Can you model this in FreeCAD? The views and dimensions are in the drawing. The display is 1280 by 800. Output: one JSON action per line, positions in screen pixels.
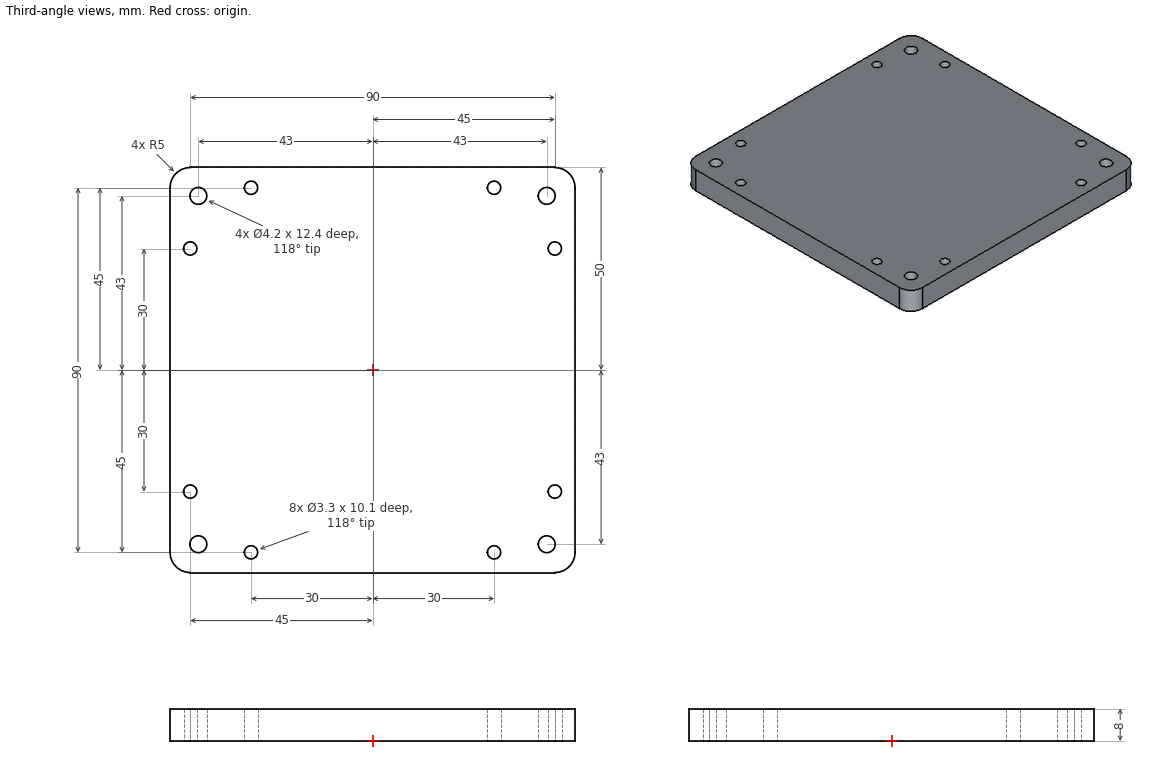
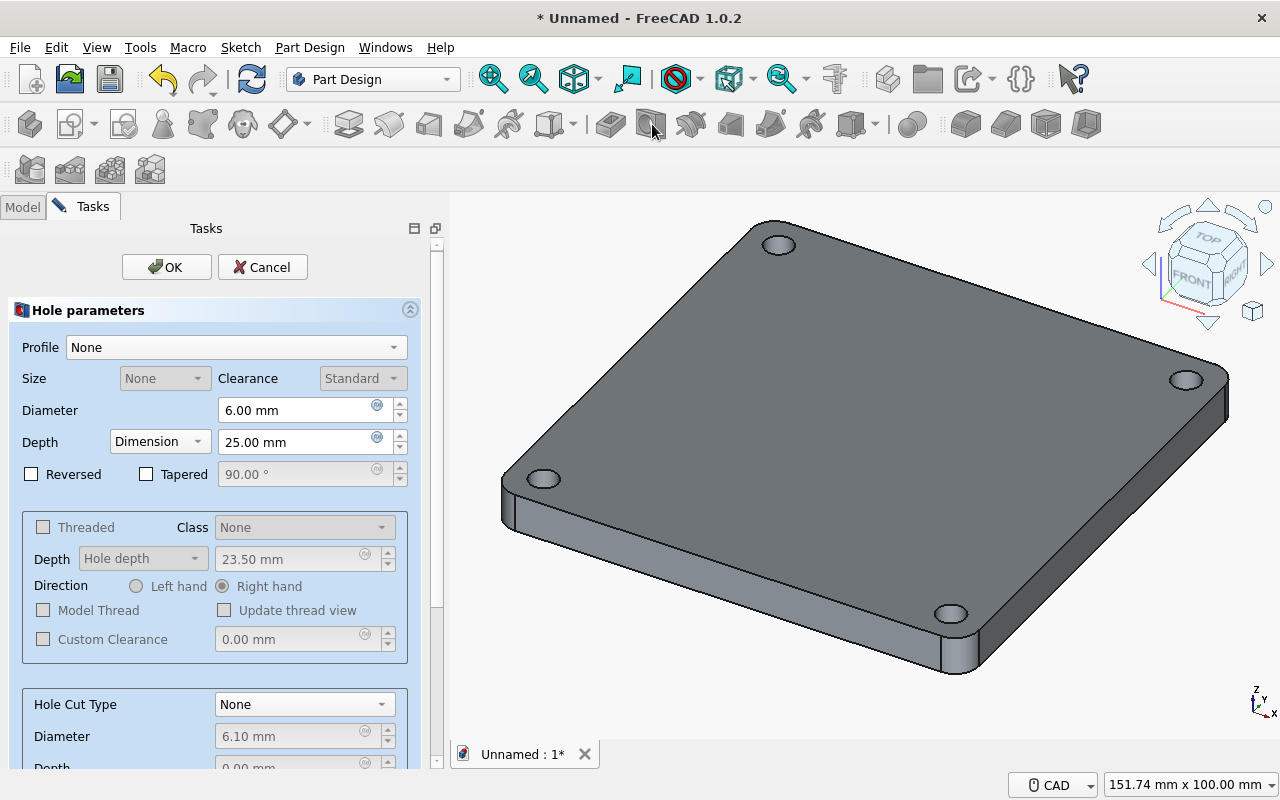
{"action": "triple_click", "coordinate": [305, 410]}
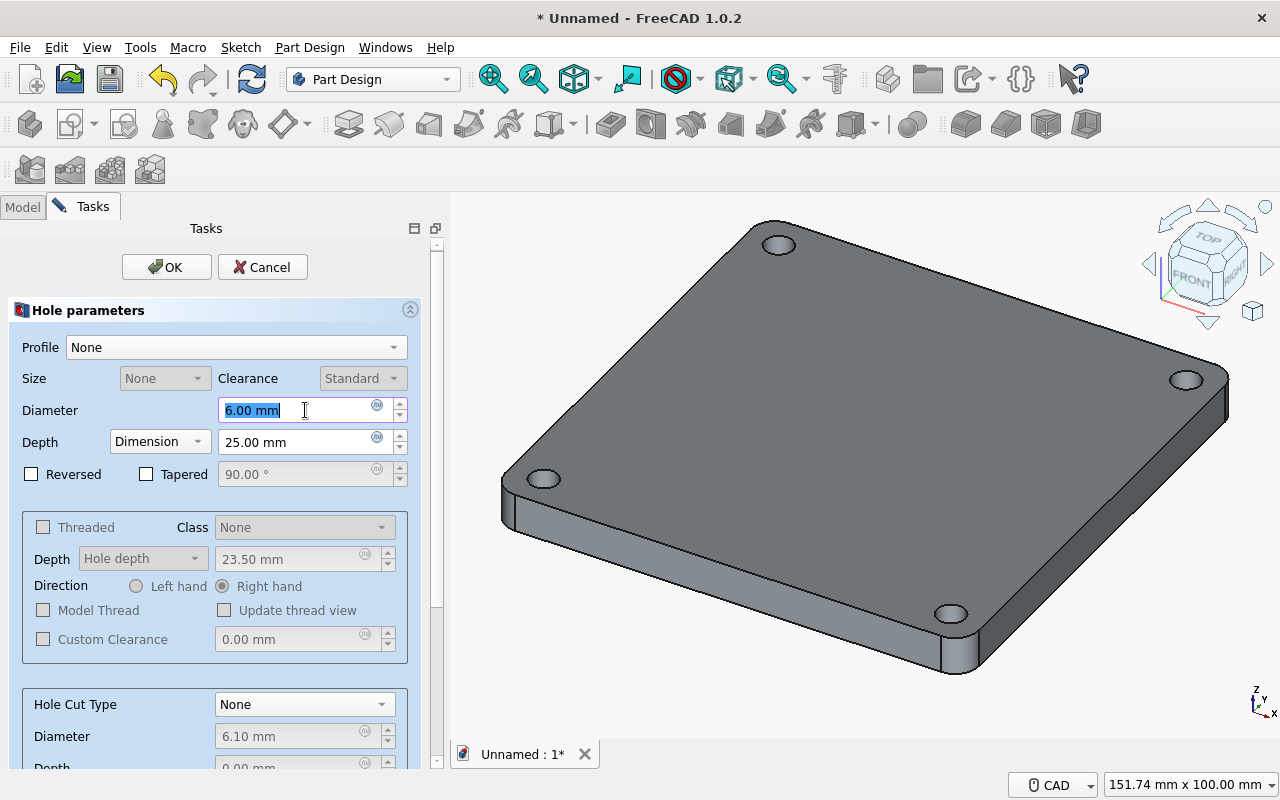
{"action": "type", "text": "4.2"}
{"action": "key", "text": "Tab"}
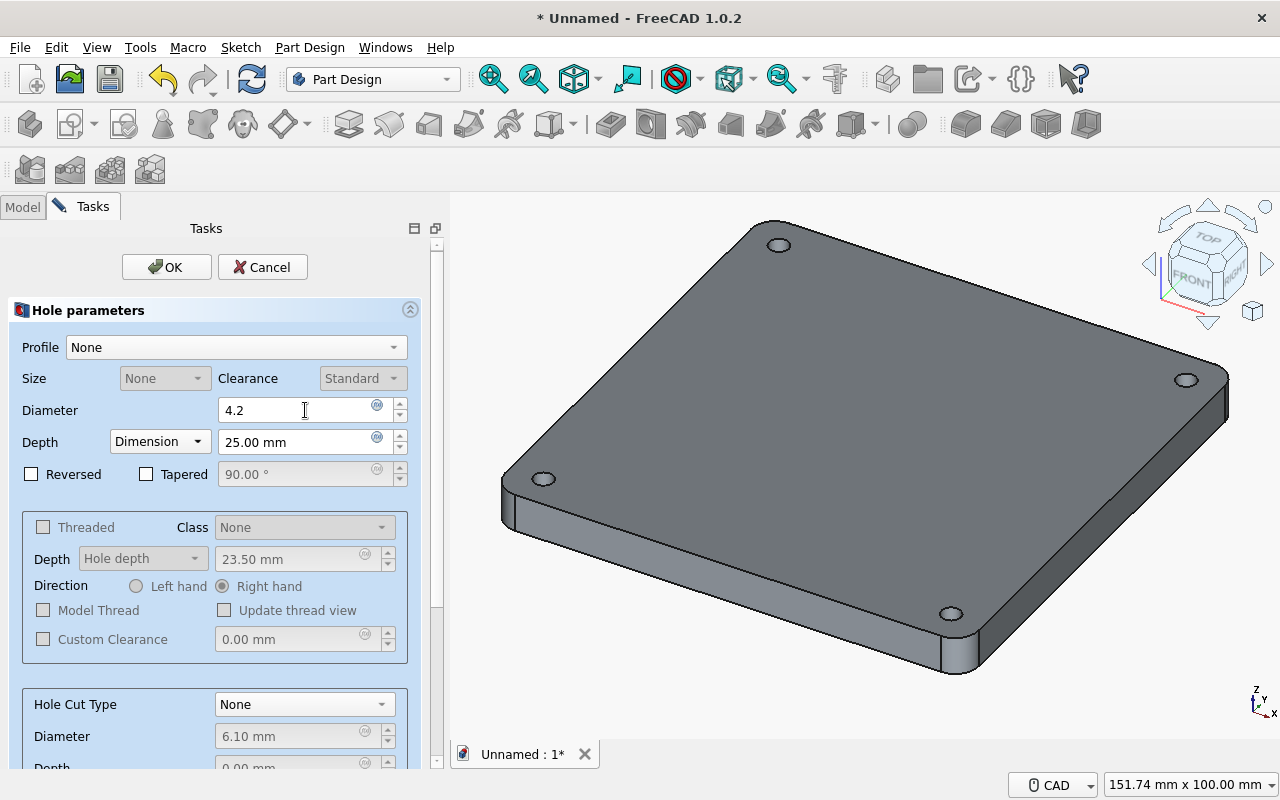
{"action": "triple_click", "coordinate": [305, 442]}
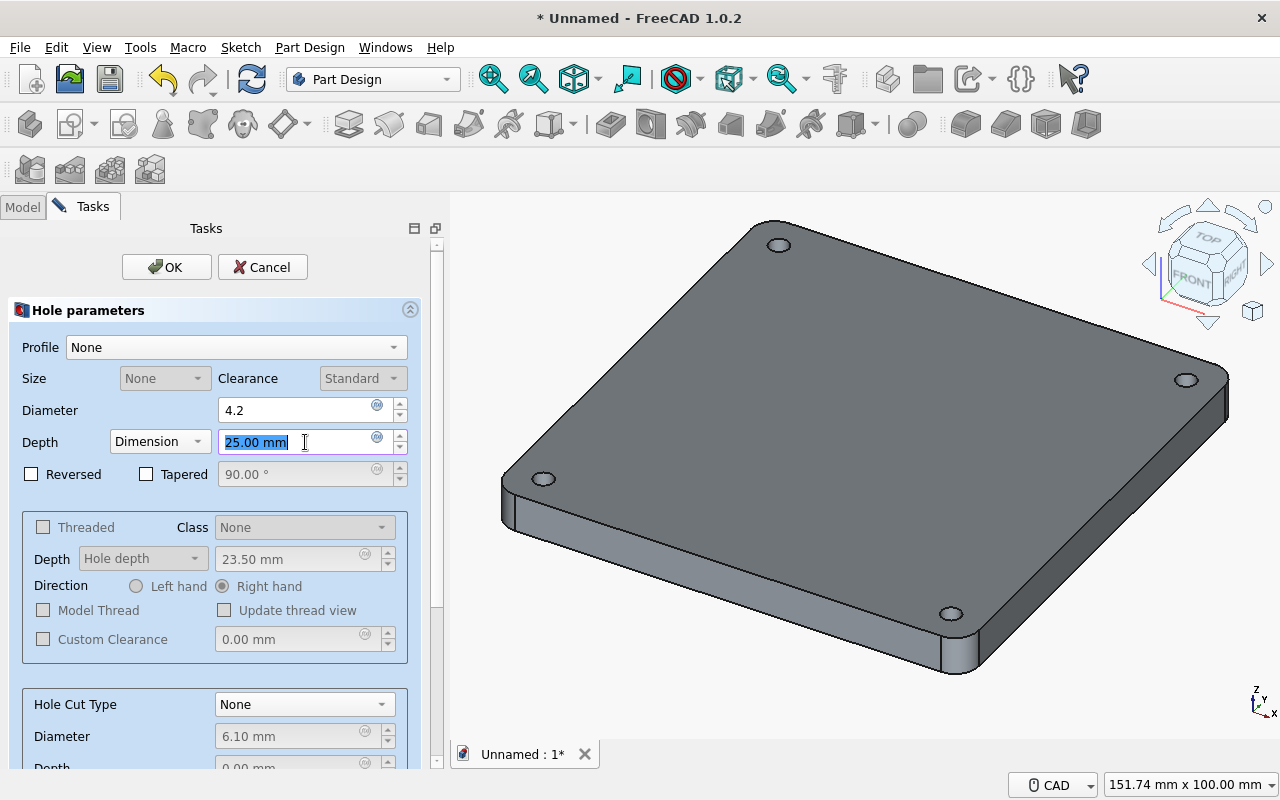
{"action": "type", "text": "12.4"}
{"action": "key", "text": "Tab"}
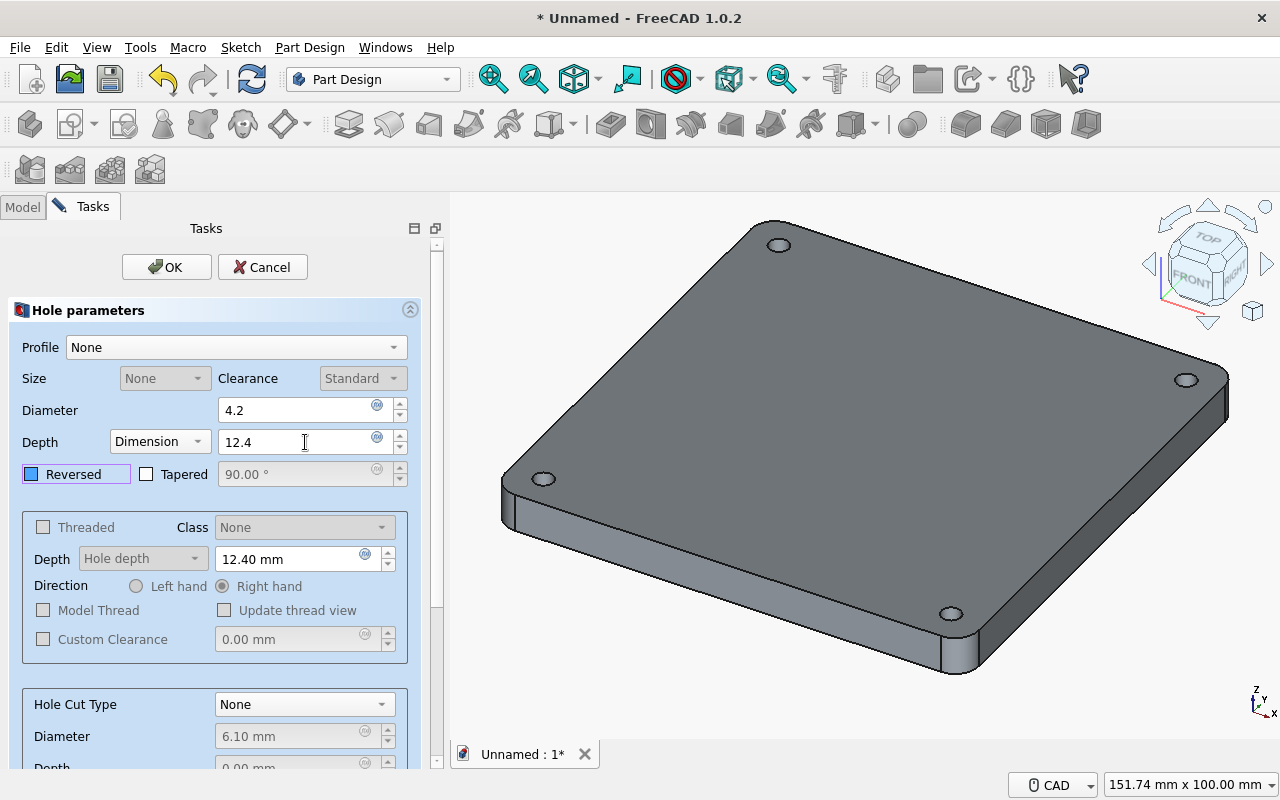
{"action": "left_click", "coordinate": [167, 267]}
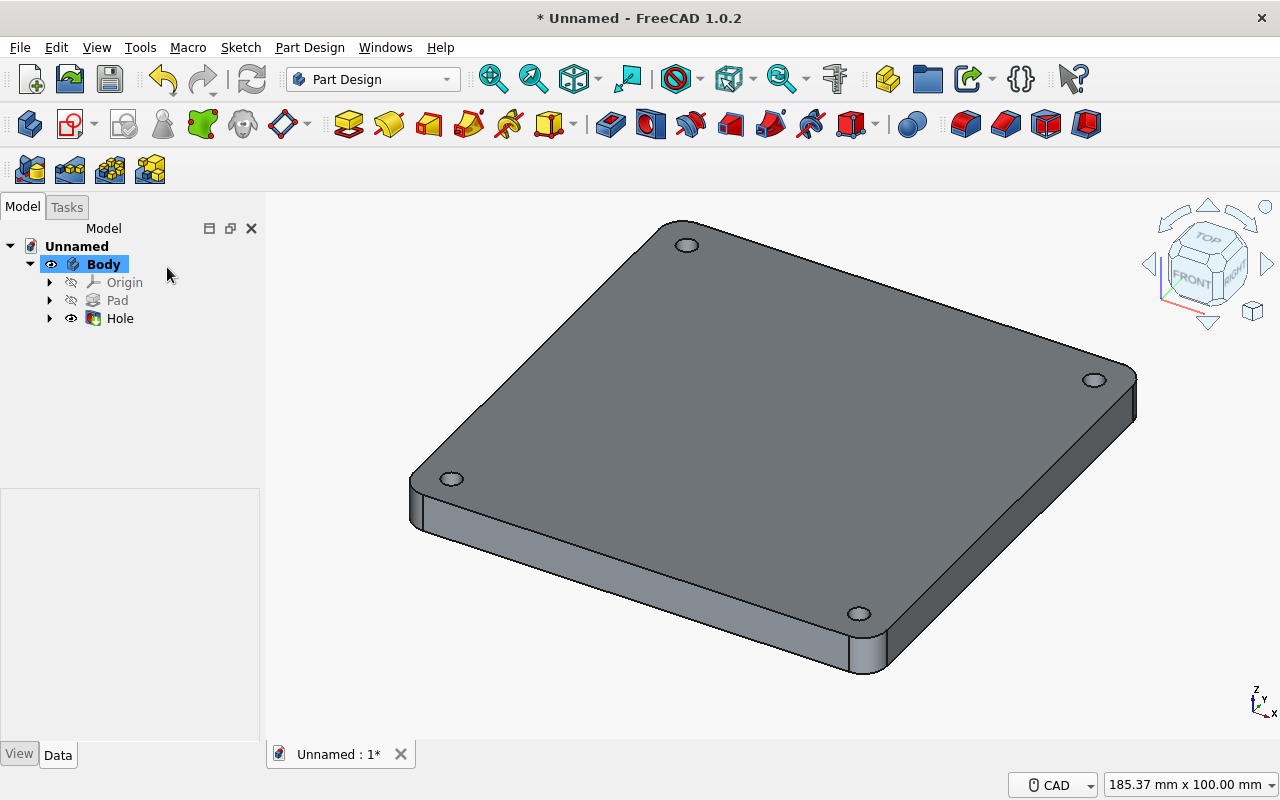
{"action": "left_click", "coordinate": [773, 429]}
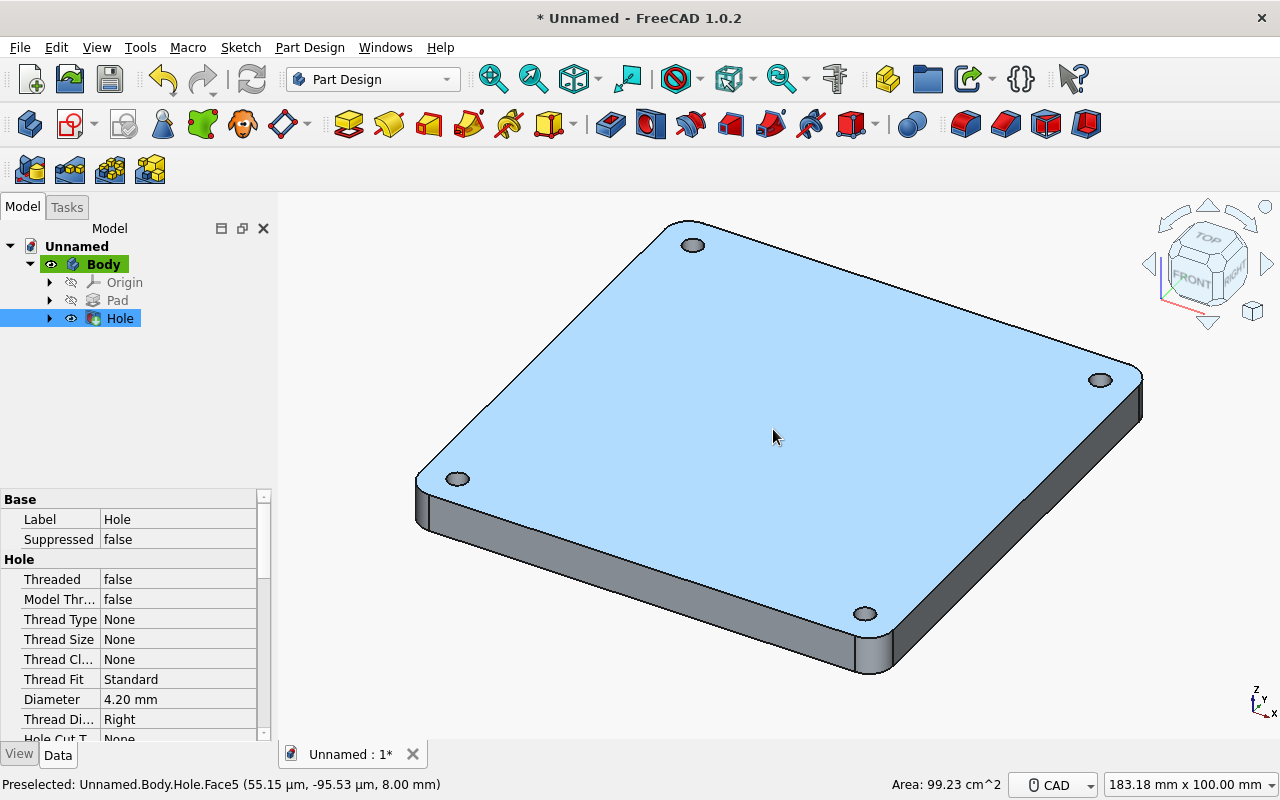
{"action": "left_click", "coordinate": [70, 124]}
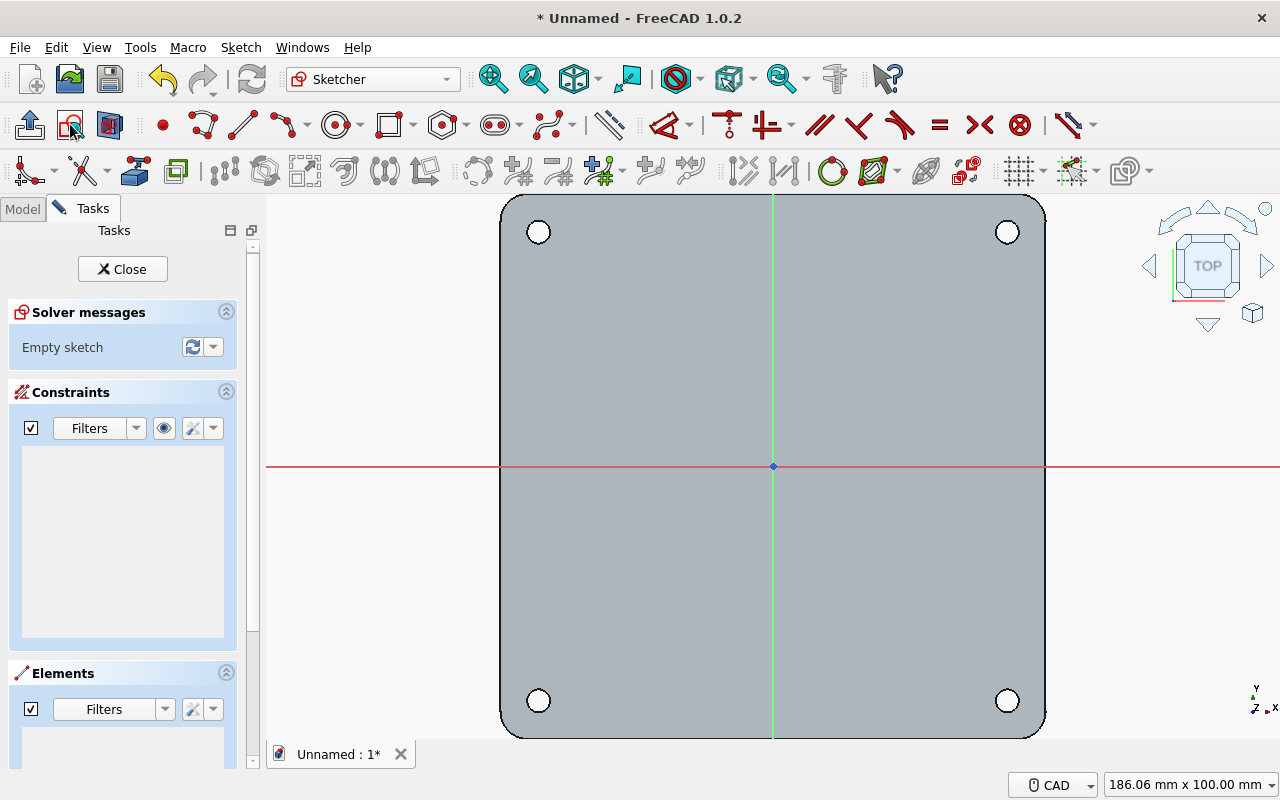
{"action": "scroll", "coordinate": [565, 466], "scroll_direction": "down", "scroll_amount": 2}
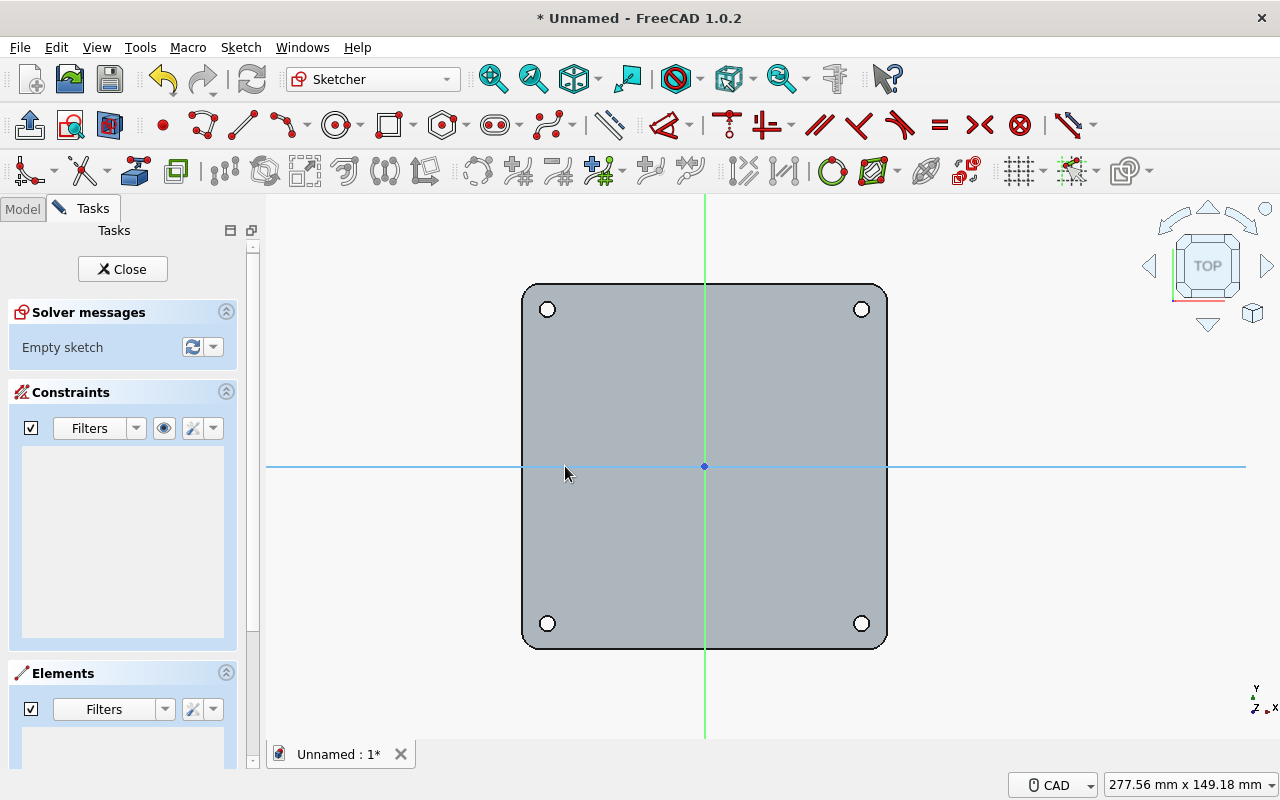
{"action": "left_click", "coordinate": [336, 126]}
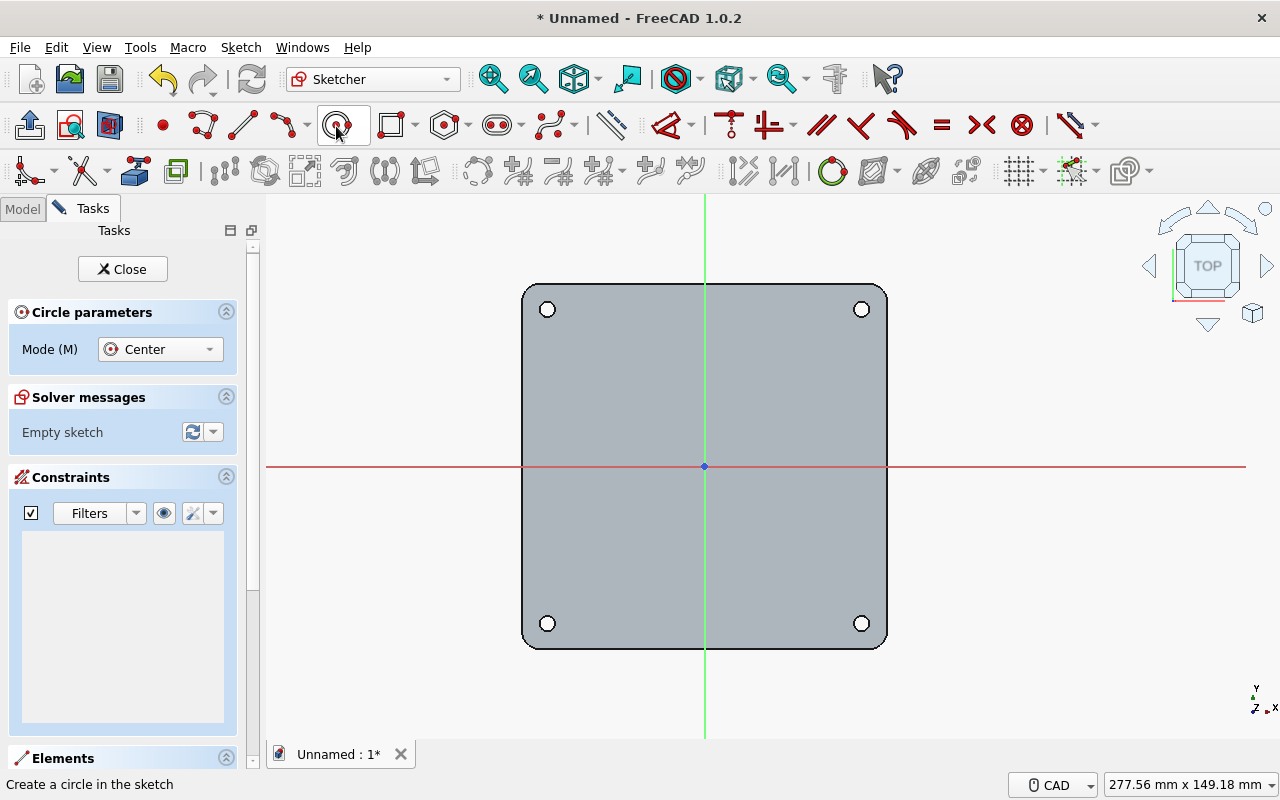
{"action": "scroll", "coordinate": [595, 631], "scroll_direction": "up", "scroll_amount": 7}